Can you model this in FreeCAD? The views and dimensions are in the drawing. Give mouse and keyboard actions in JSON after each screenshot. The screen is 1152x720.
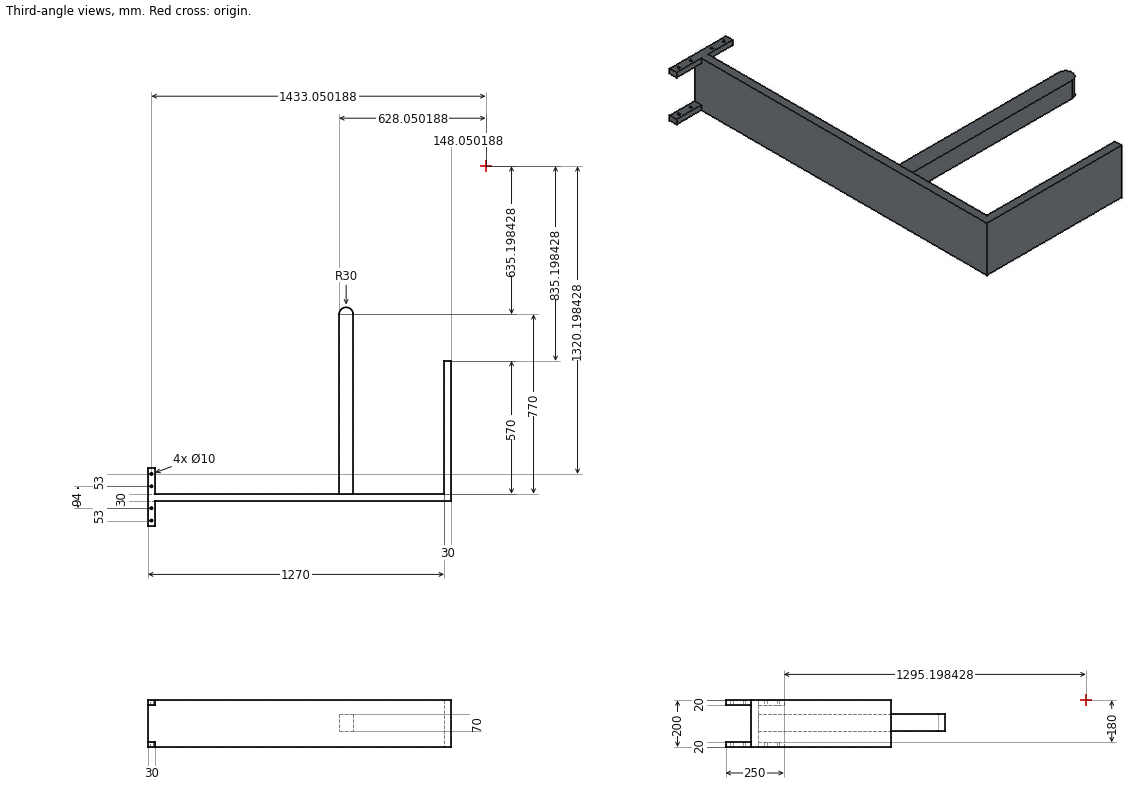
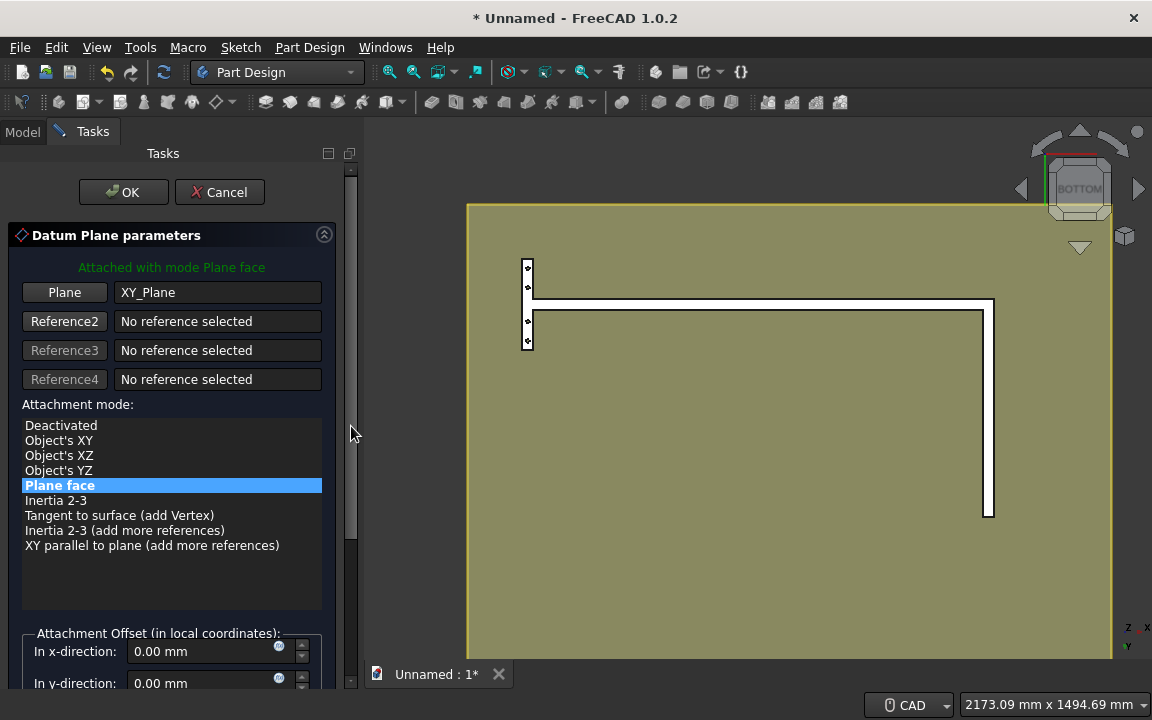
{"action": "left_click", "coordinate": [124, 192]}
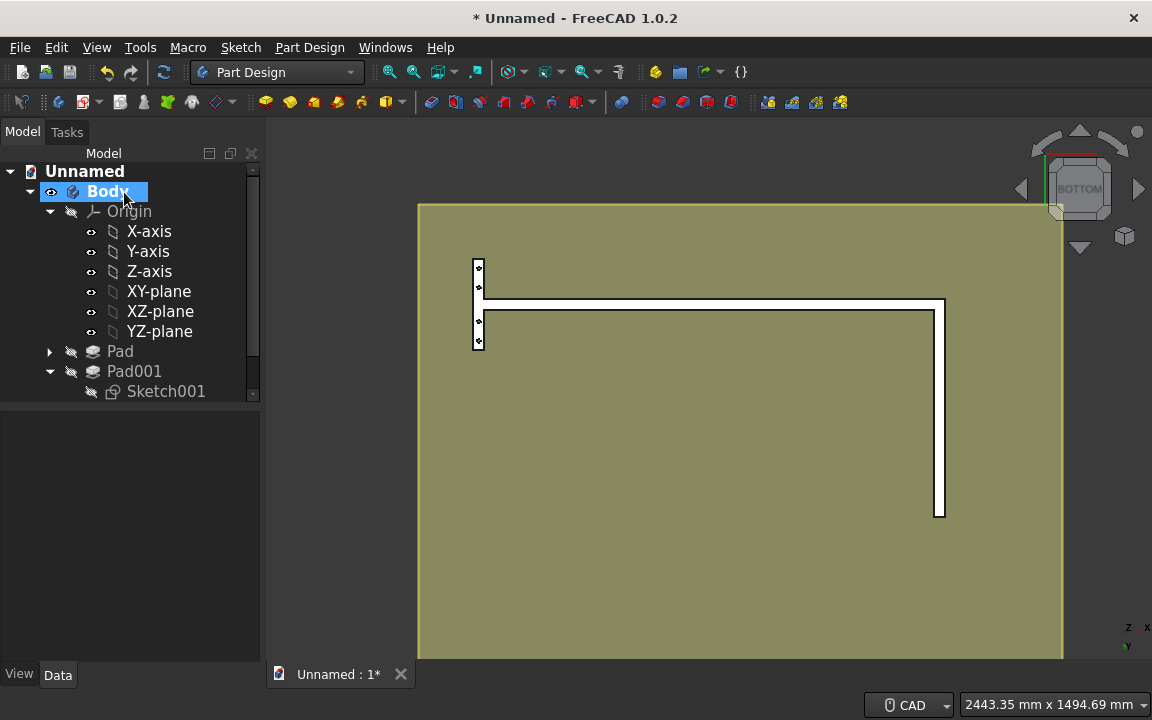
{"action": "scroll", "coordinate": [100, 287], "scroll_direction": "down", "scroll_amount": 3}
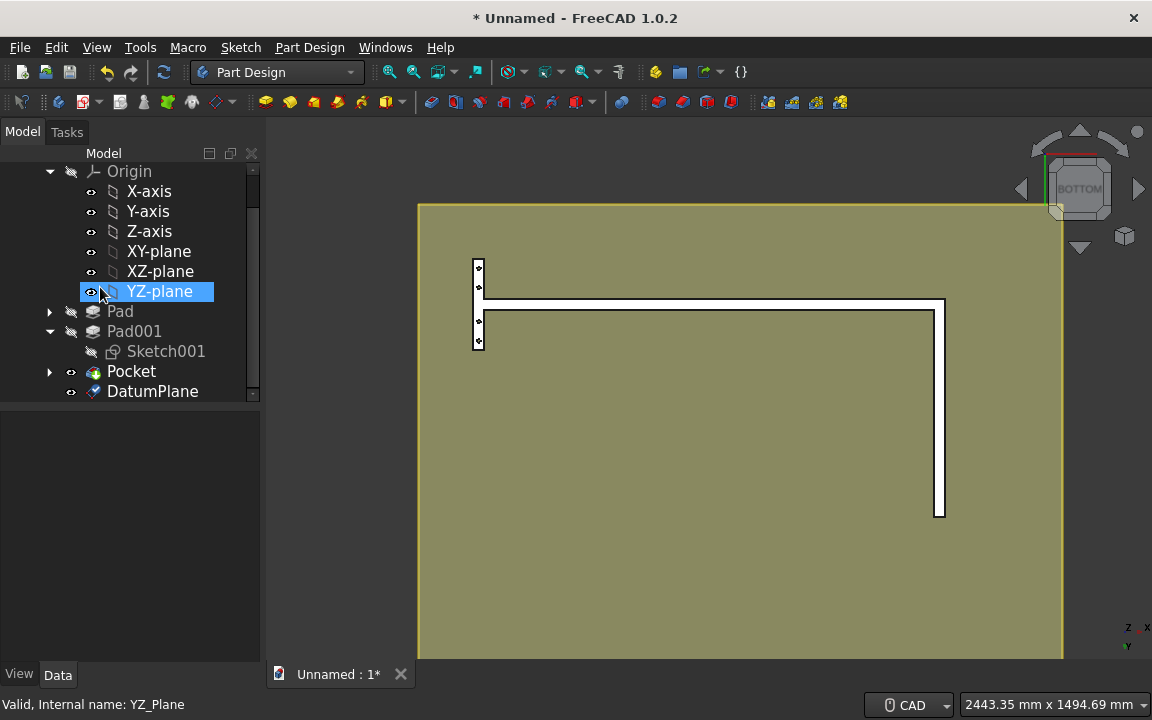
{"action": "left_click", "coordinate": [116, 392]}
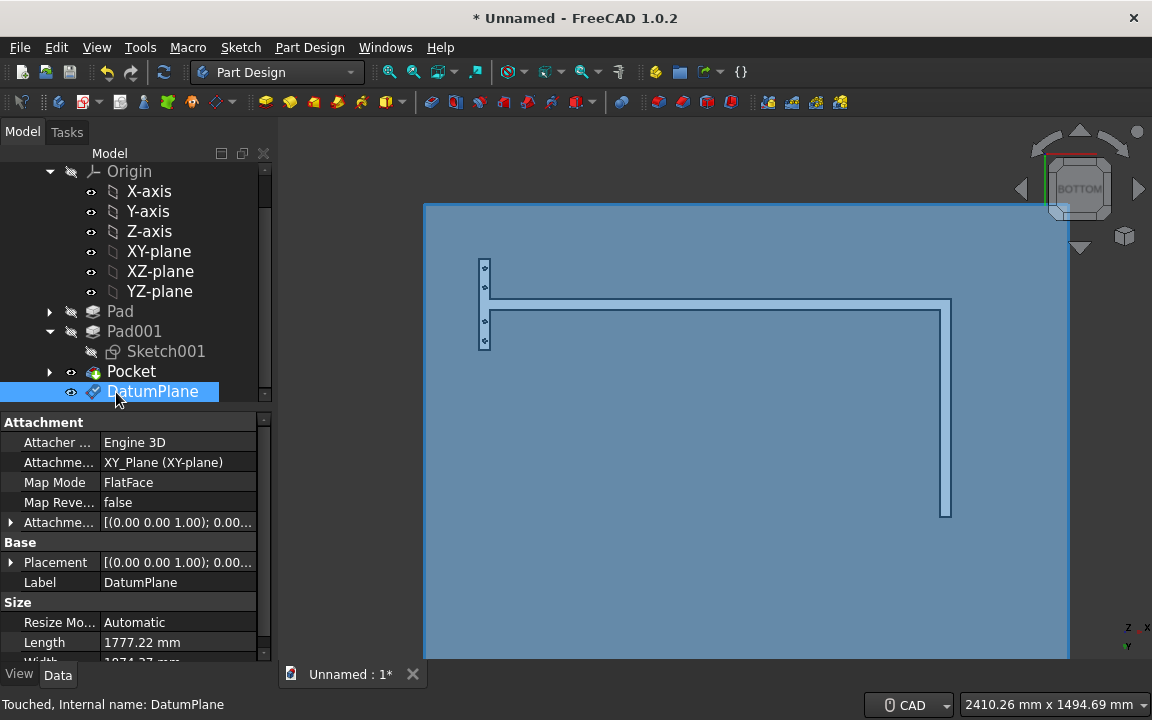
{"action": "left_click", "coordinate": [84, 102]}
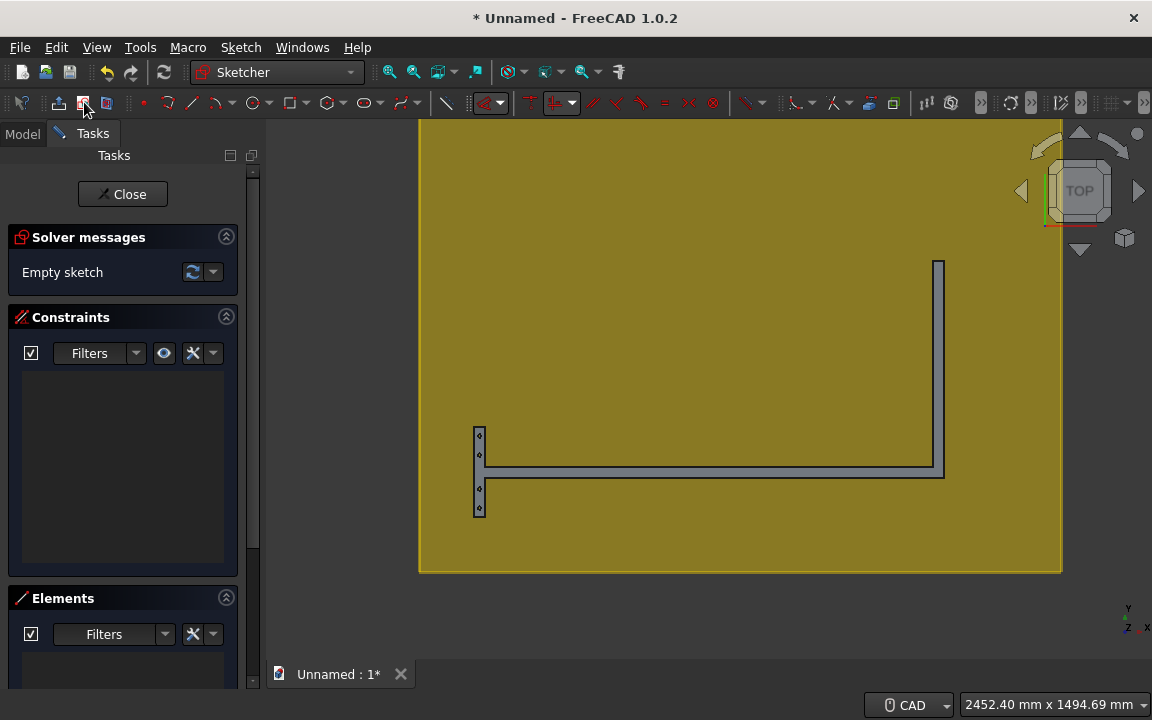
{"action": "left_click", "coordinate": [108, 104]}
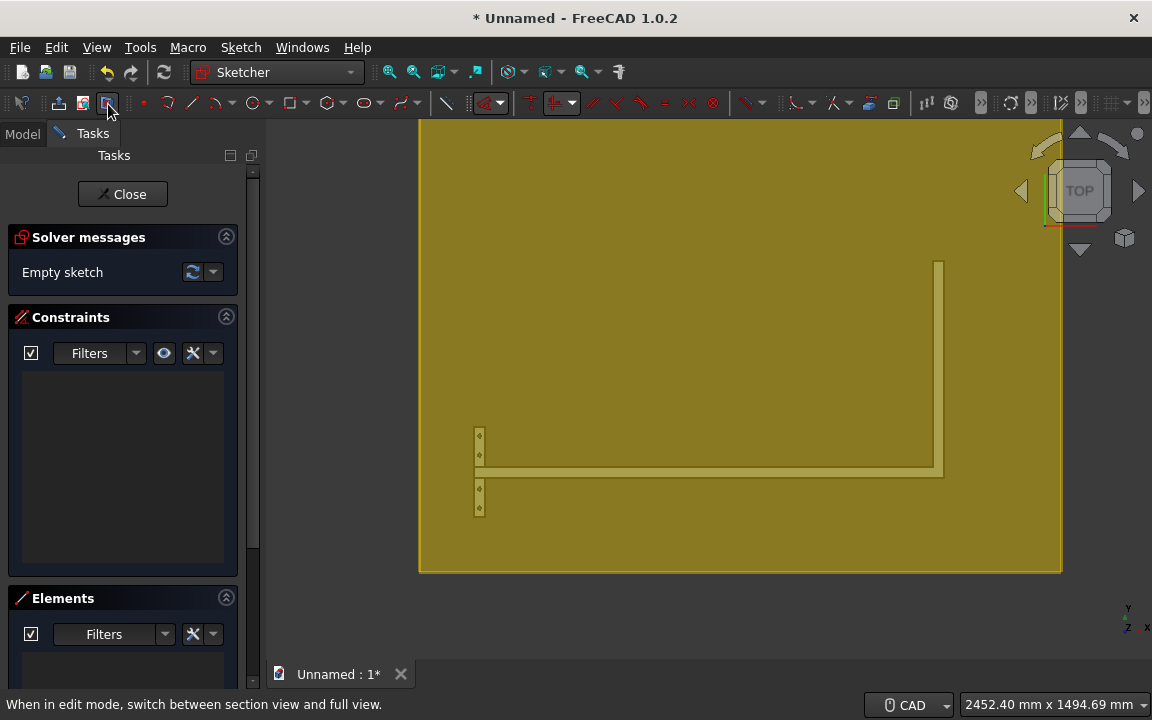
{"action": "scroll", "coordinate": [294, 631], "scroll_direction": "down", "scroll_amount": 2}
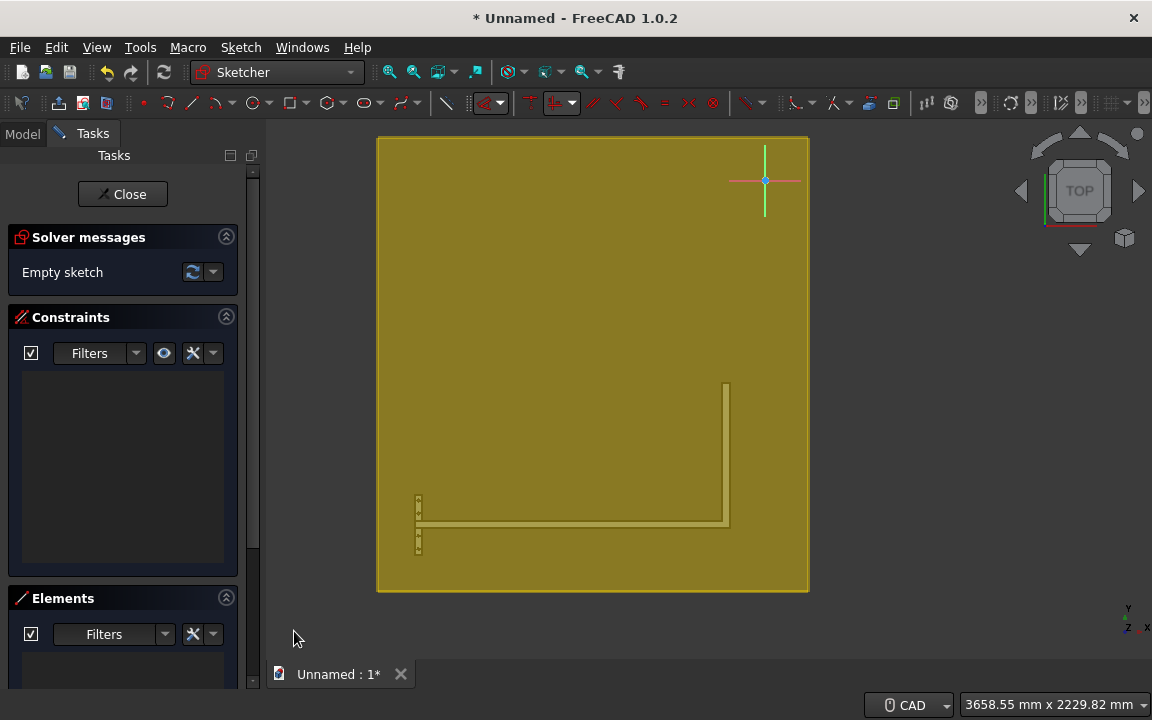
{"action": "left_click", "coordinate": [168, 104]}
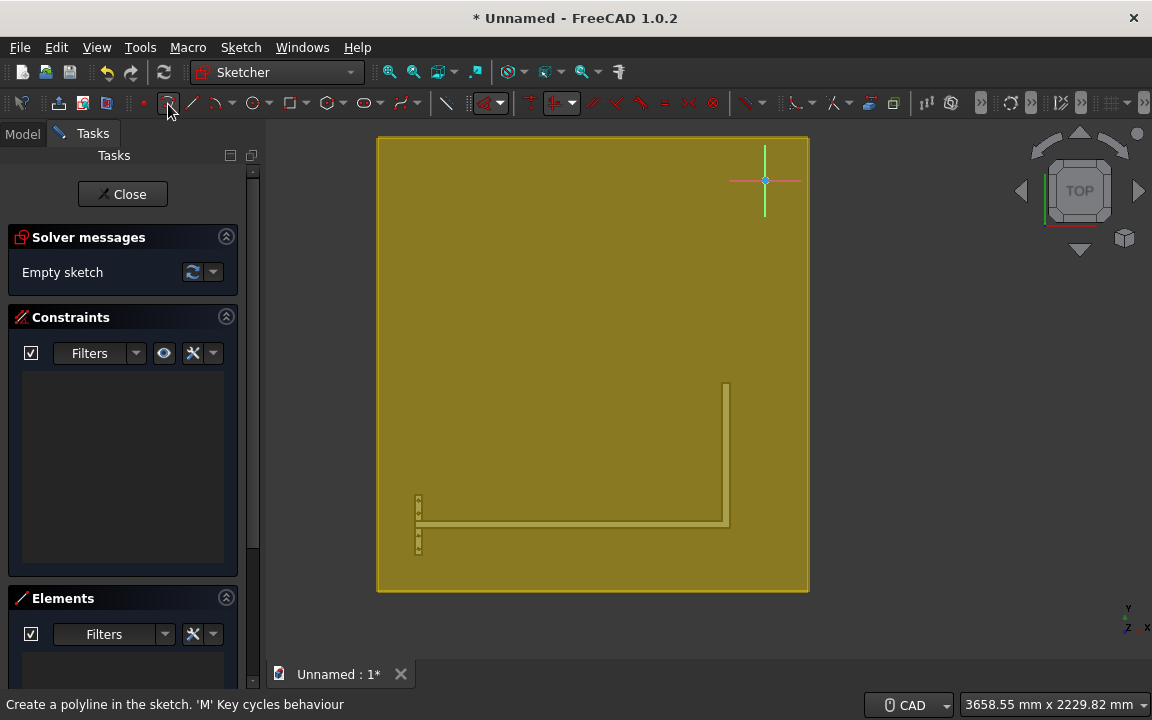
{"action": "left_click", "coordinate": [613, 335]}
{"action": "left_click", "coordinate": [613, 521]}
{"action": "left_click", "coordinate": [628, 521]}
{"action": "left_click", "coordinate": [628, 335]}
{"action": "right_click", "coordinate": [628, 335]}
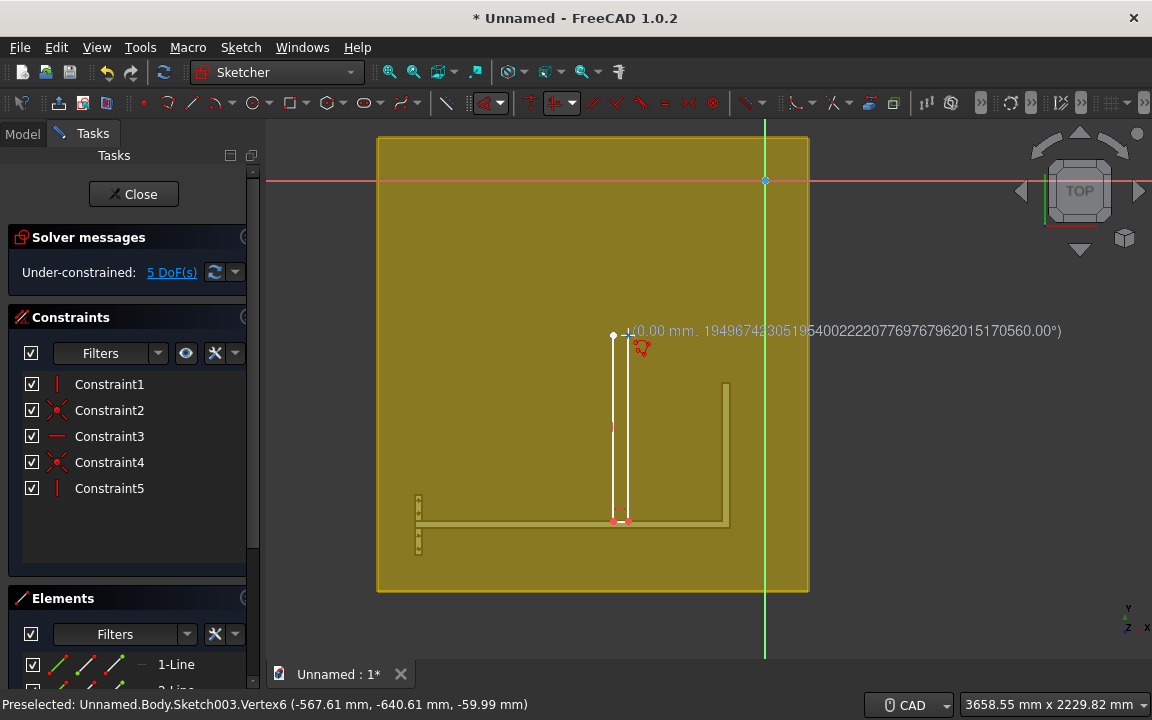
{"action": "left_click", "coordinate": [234, 104]}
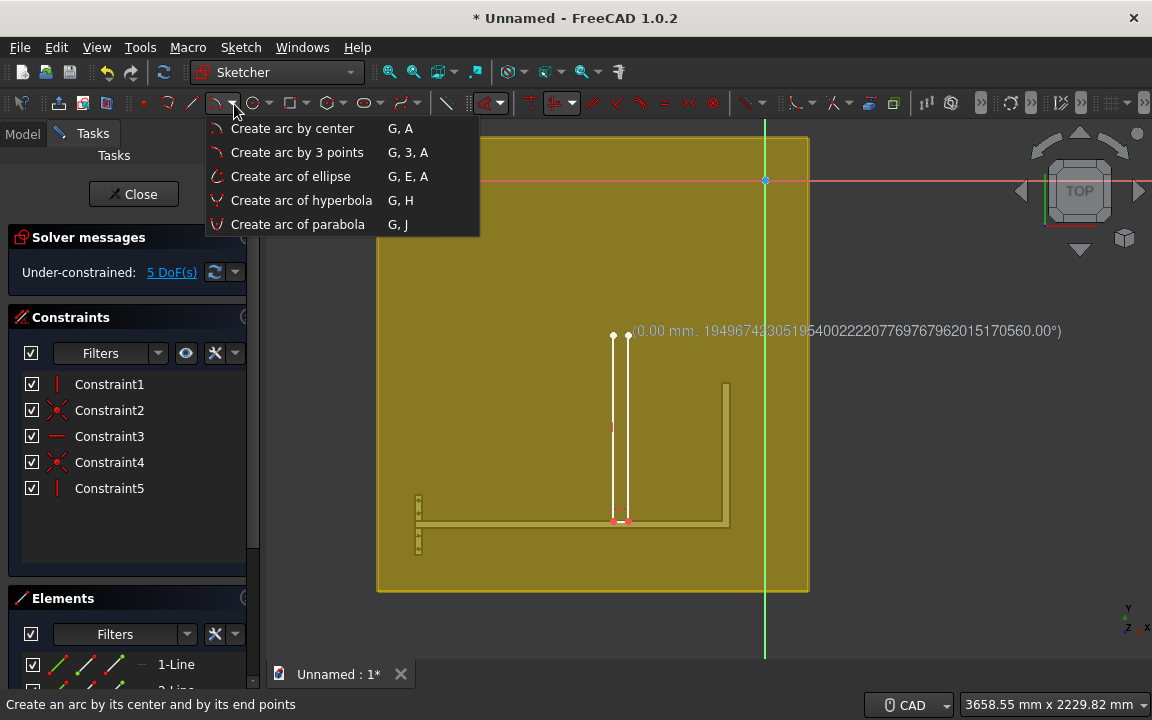
{"action": "left_click", "coordinate": [342, 152]}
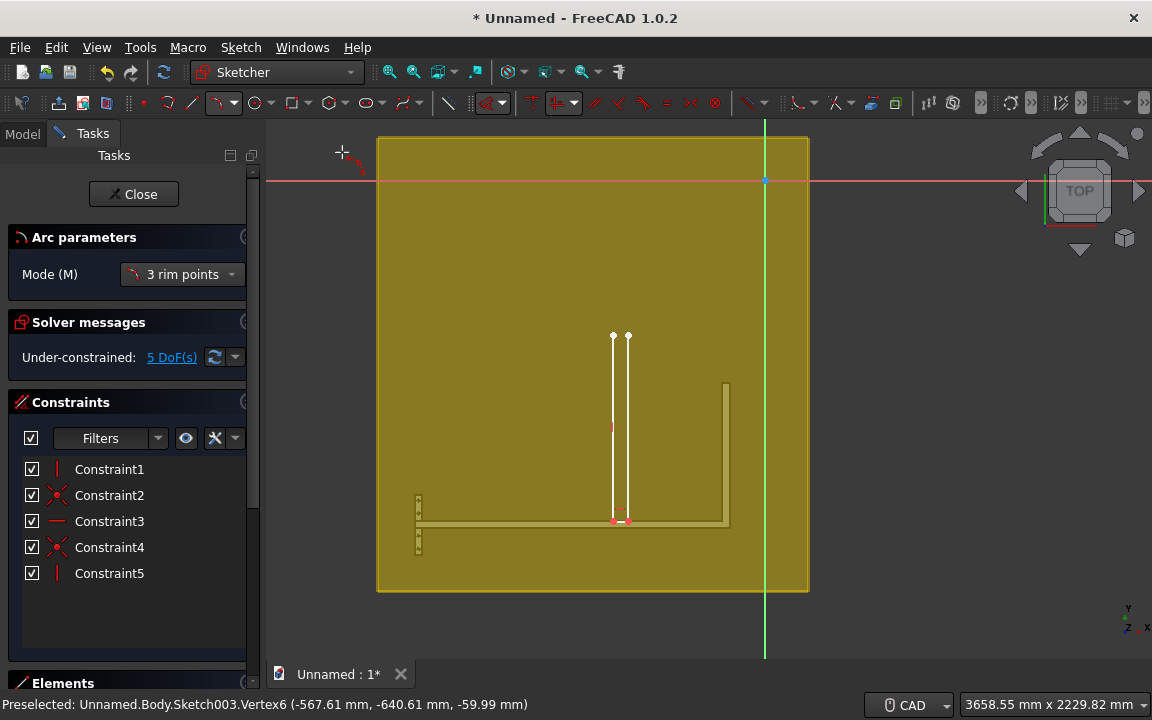
{"action": "left_click", "coordinate": [628, 336]}
{"action": "left_click", "coordinate": [613, 336]}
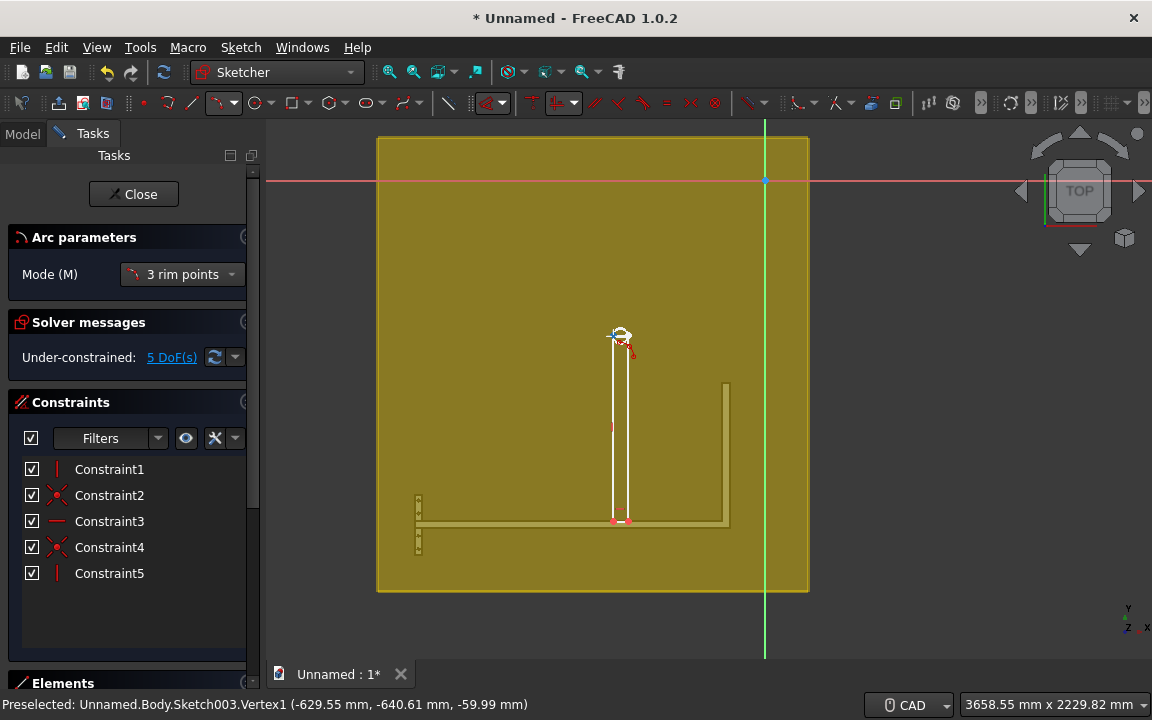
{"action": "scroll", "coordinate": [621, 327], "scroll_direction": "up", "scroll_amount": 4}